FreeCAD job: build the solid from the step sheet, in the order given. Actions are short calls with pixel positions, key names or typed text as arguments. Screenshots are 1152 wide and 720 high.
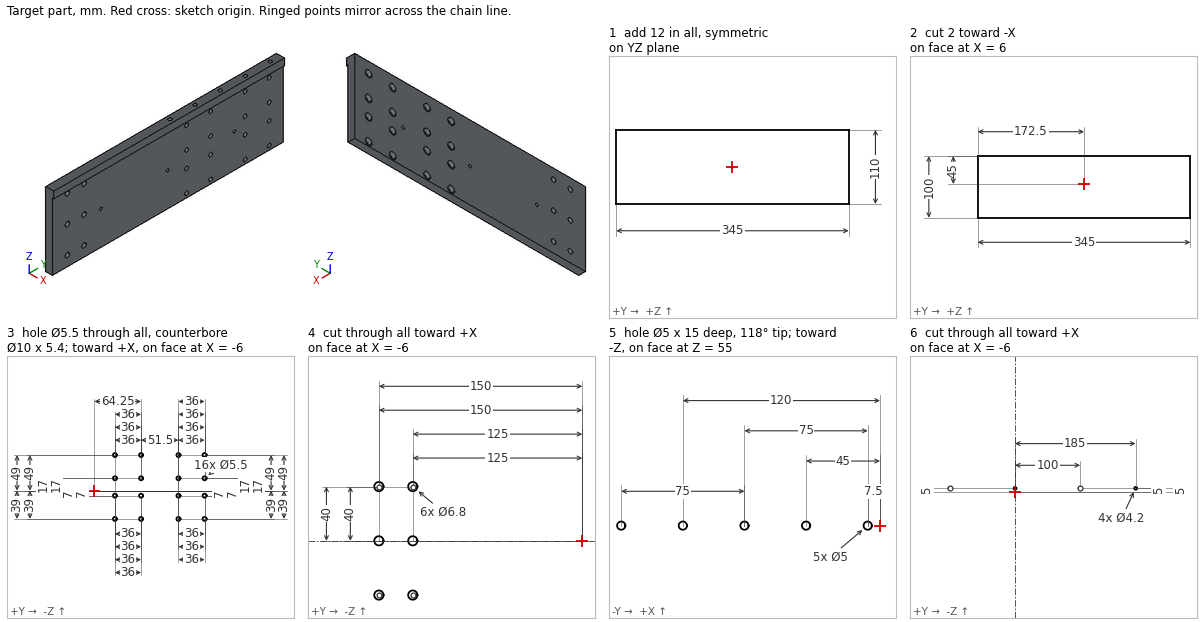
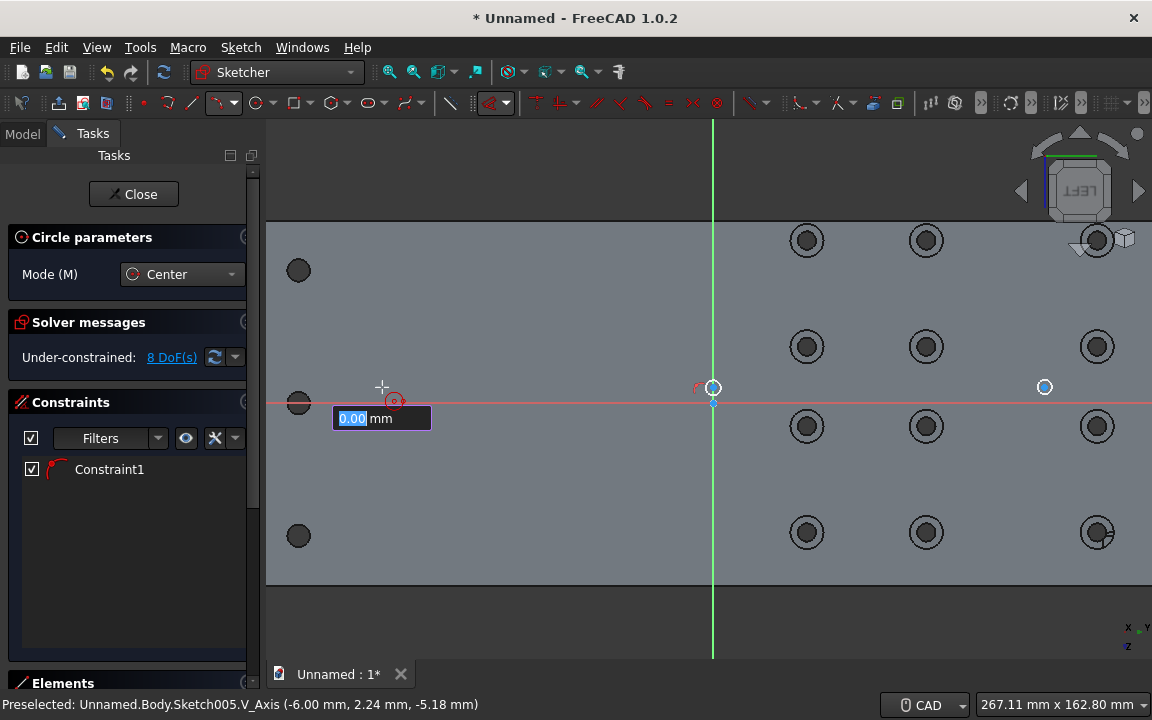
scroll(386, 382, up, 5)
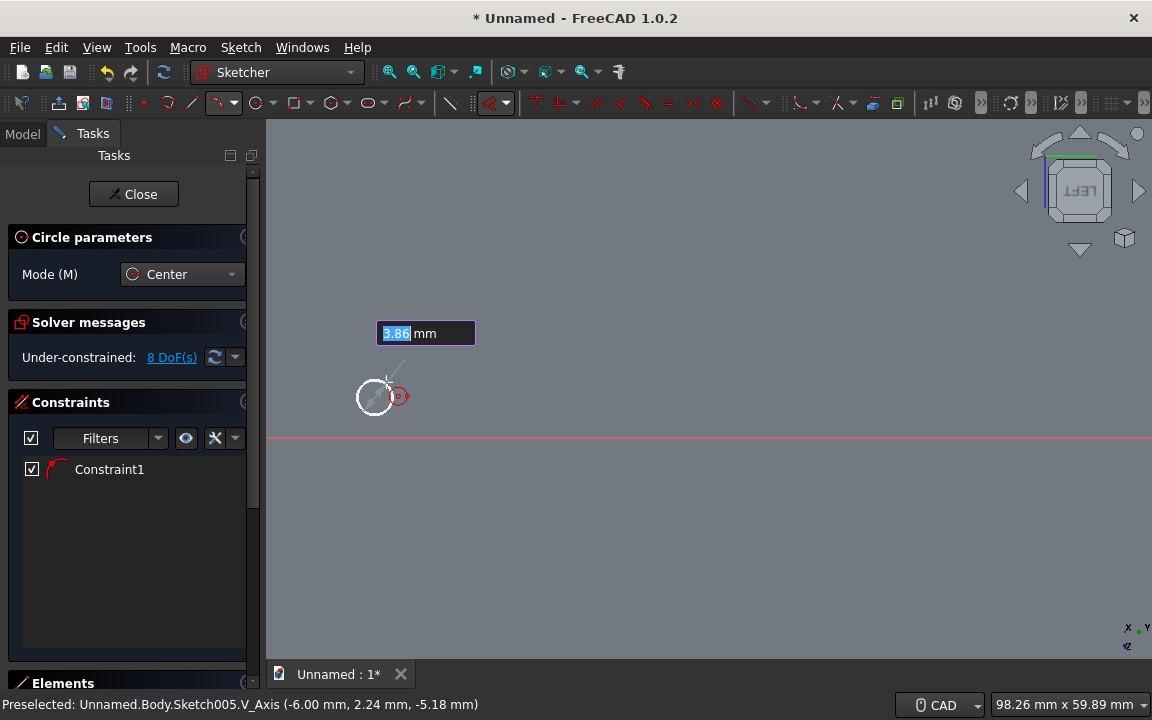
click(387, 380)
key(Escape)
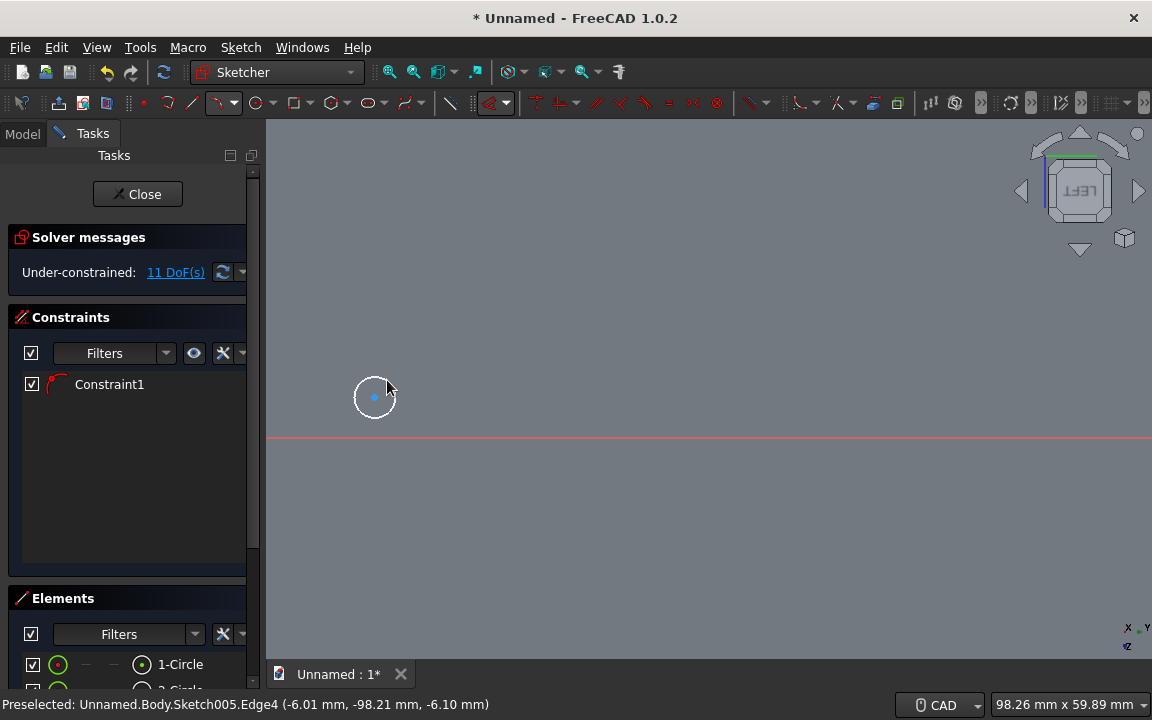
scroll(383, 385, down, 8)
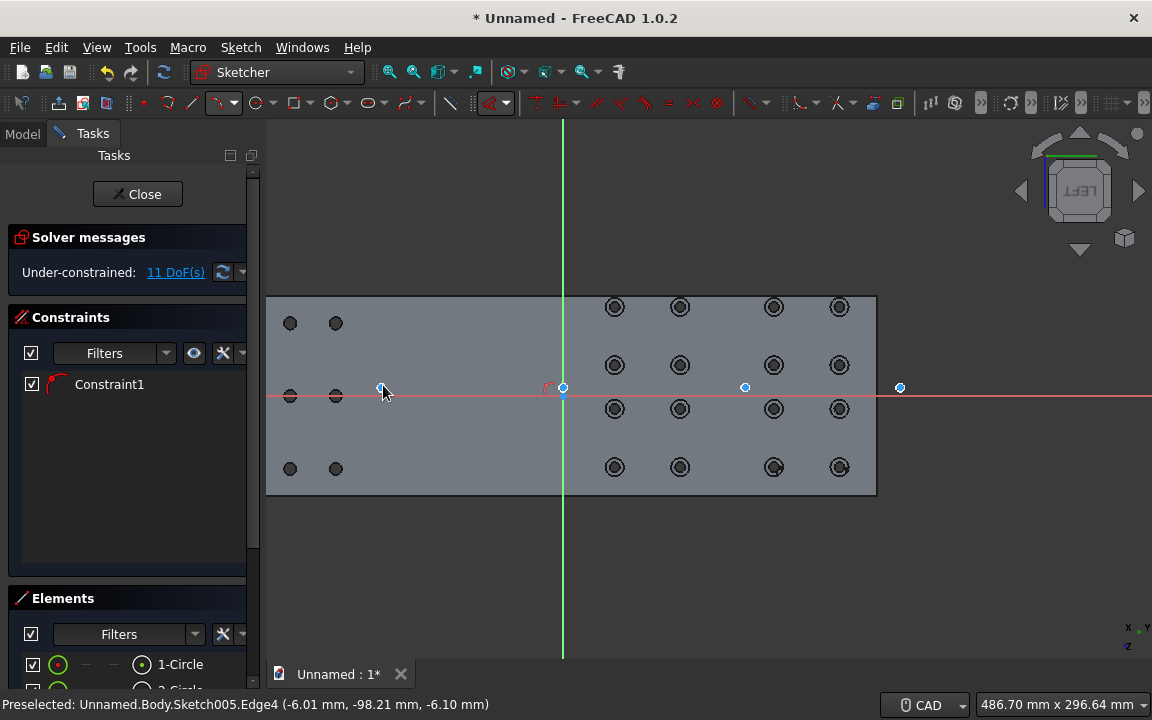
scroll(903, 385, up, 7)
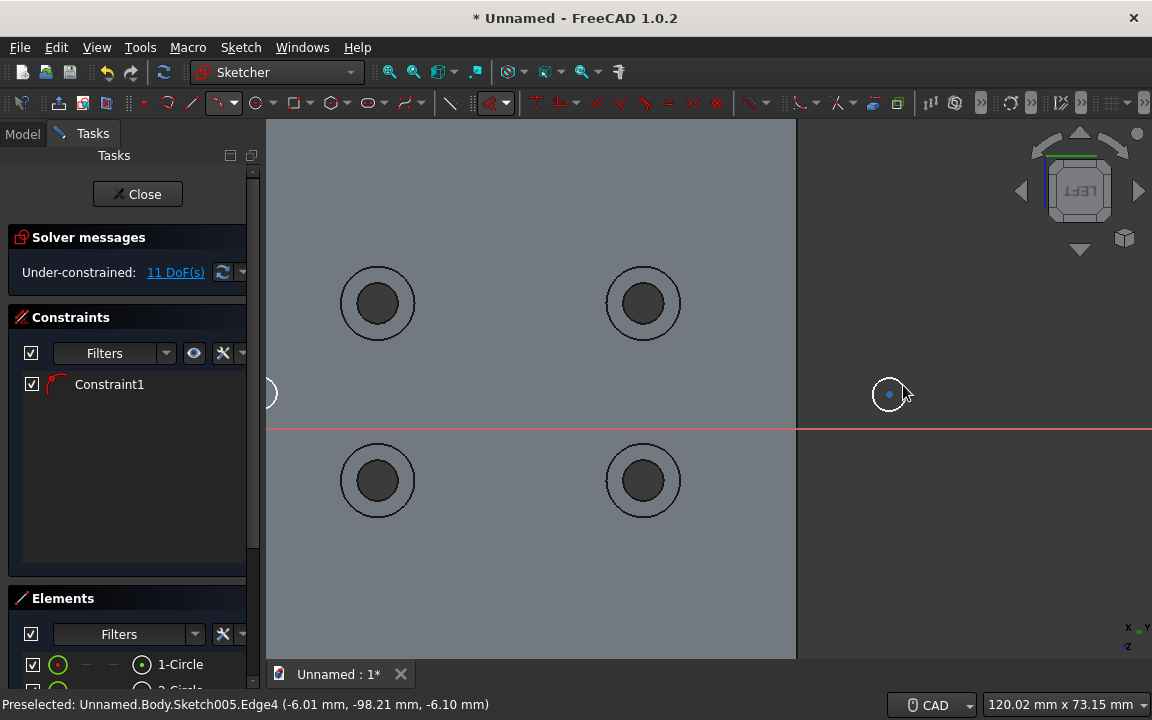
click(901, 383)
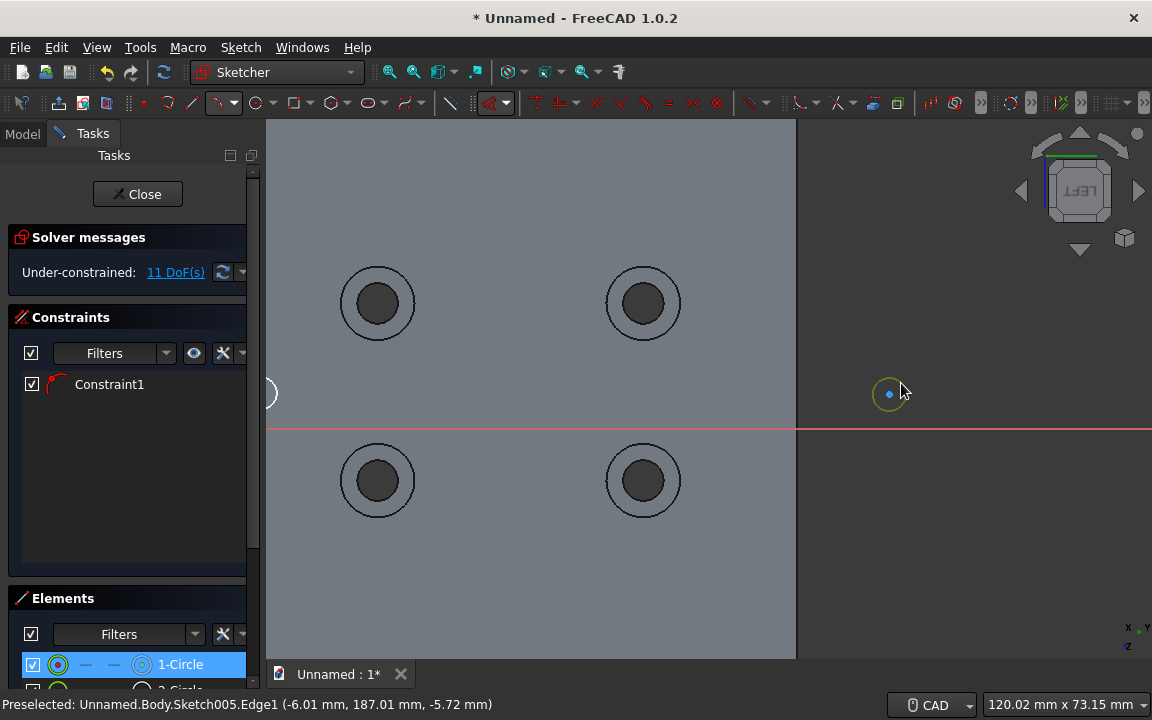
scroll(904, 385, down, 7)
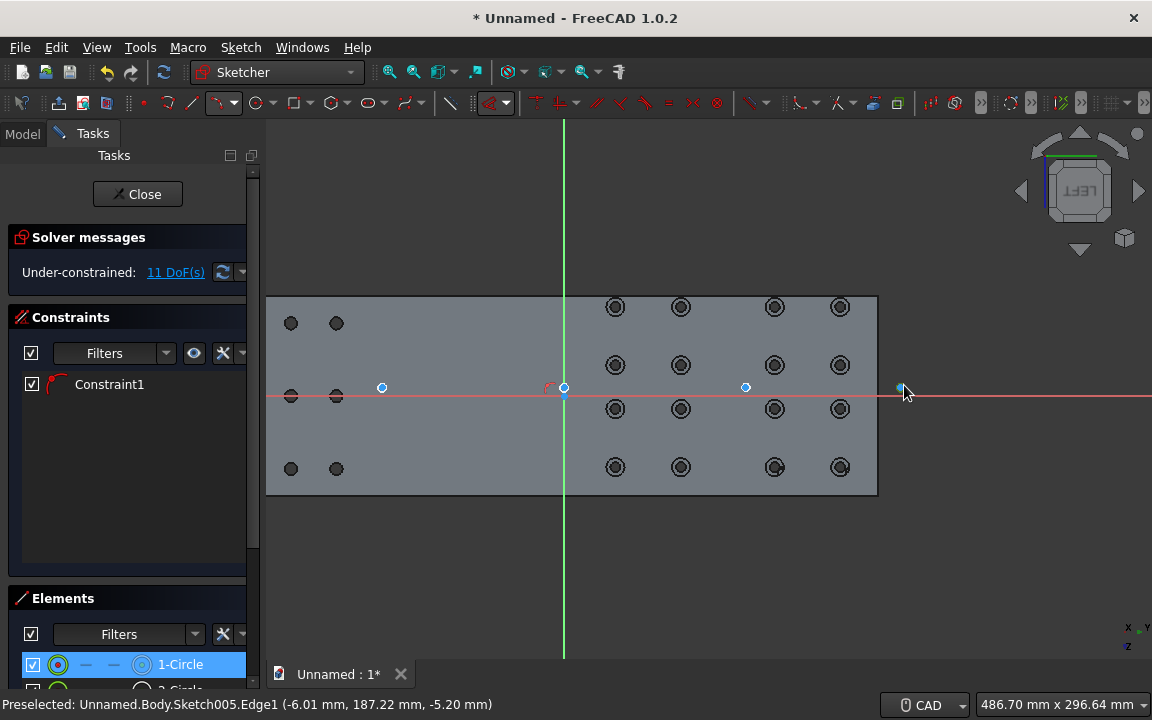
scroll(749, 385, up, 7)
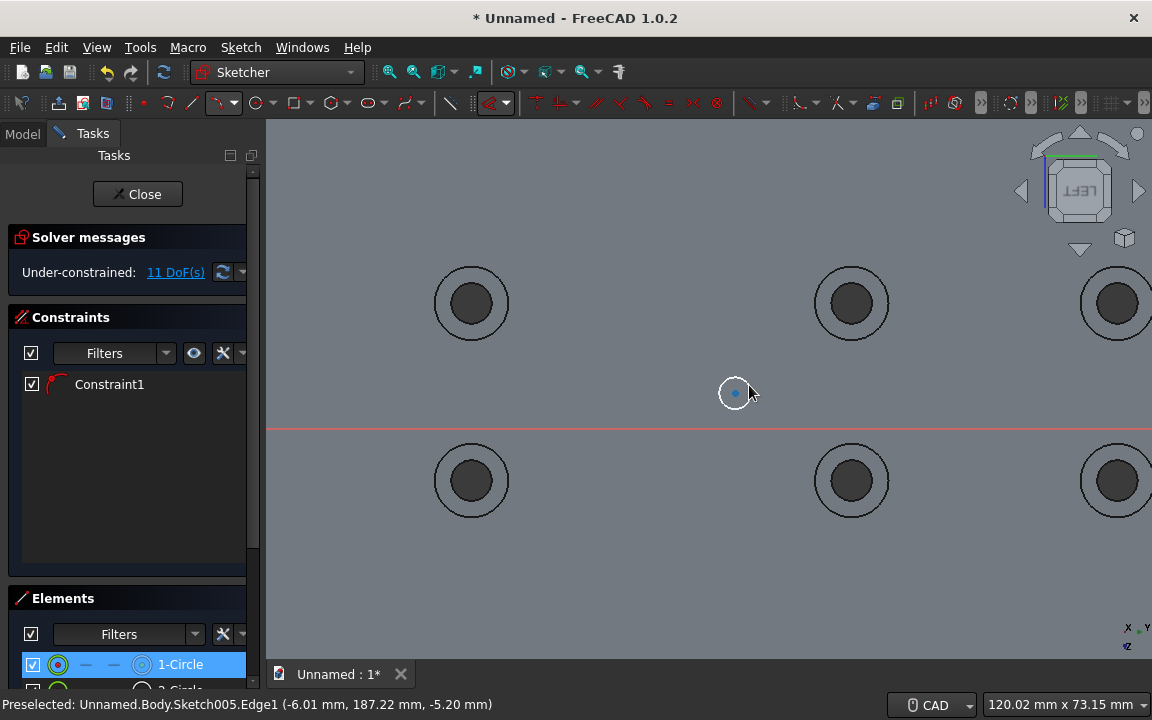
click(746, 382)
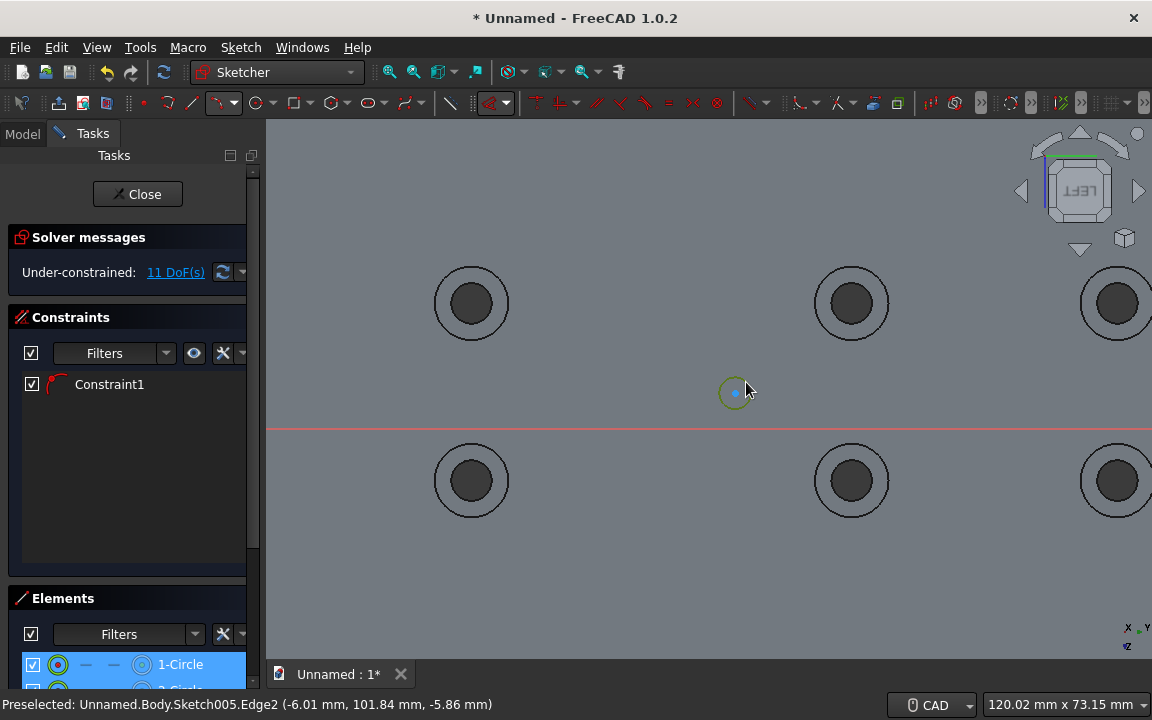
scroll(748, 385, down, 7)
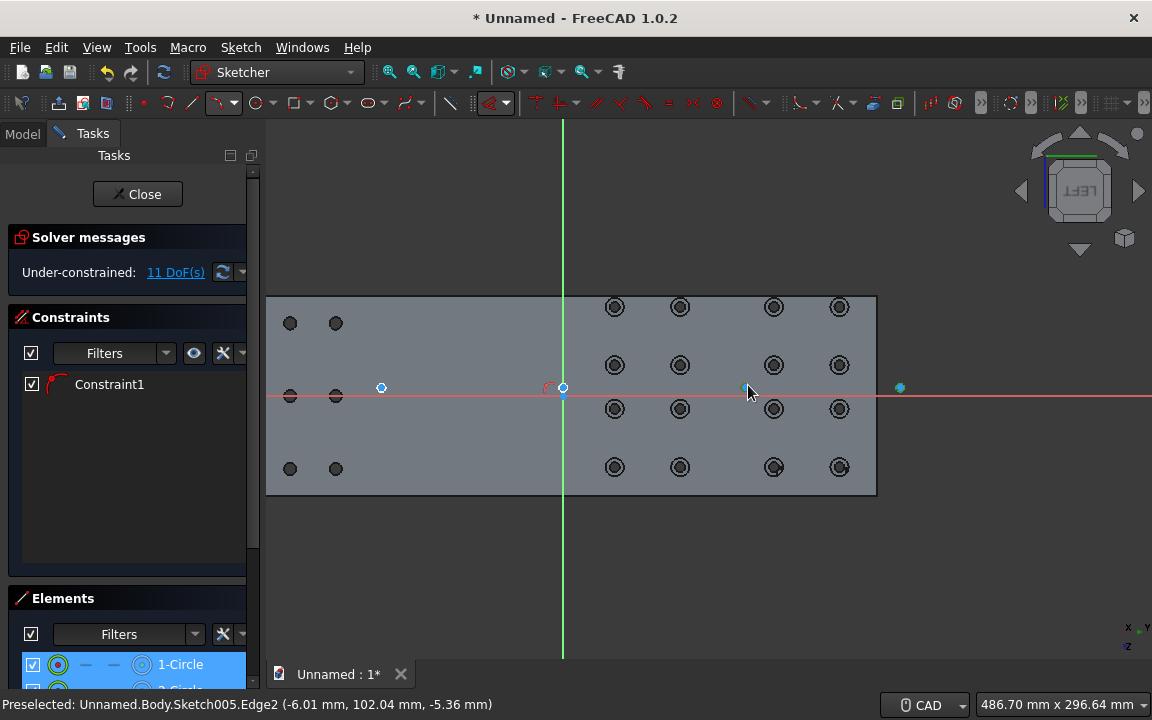
scroll(566, 385, up, 8)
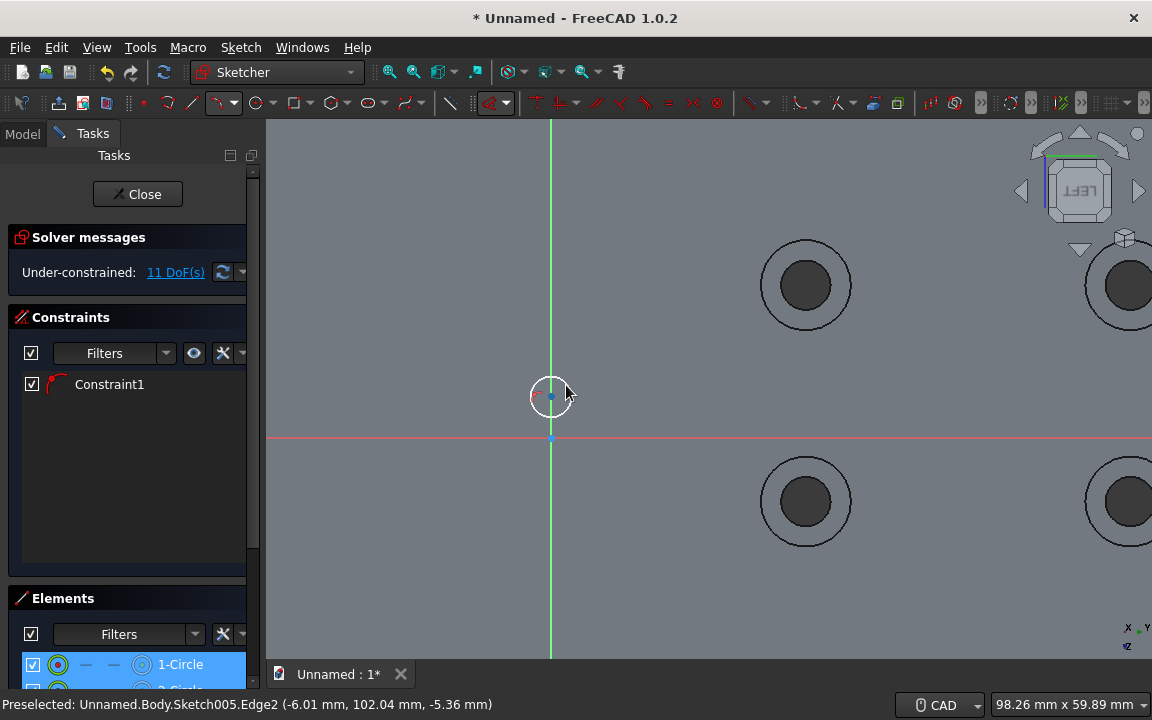
click(565, 383)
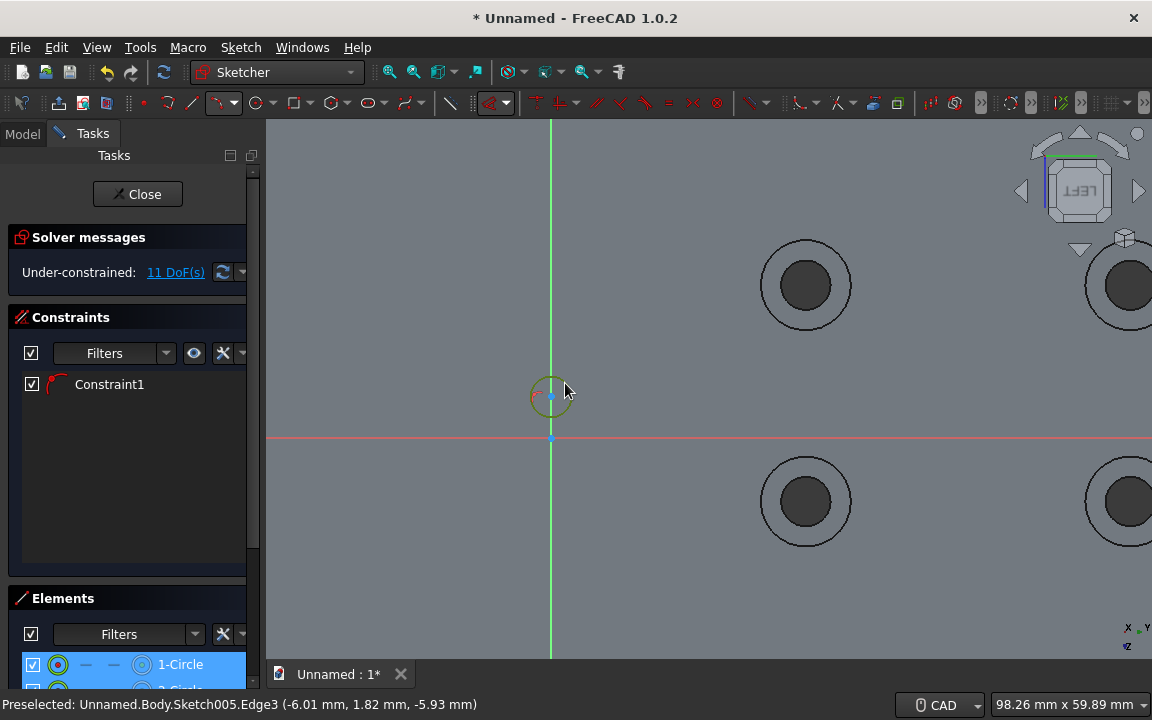
scroll(566, 385, down, 8)